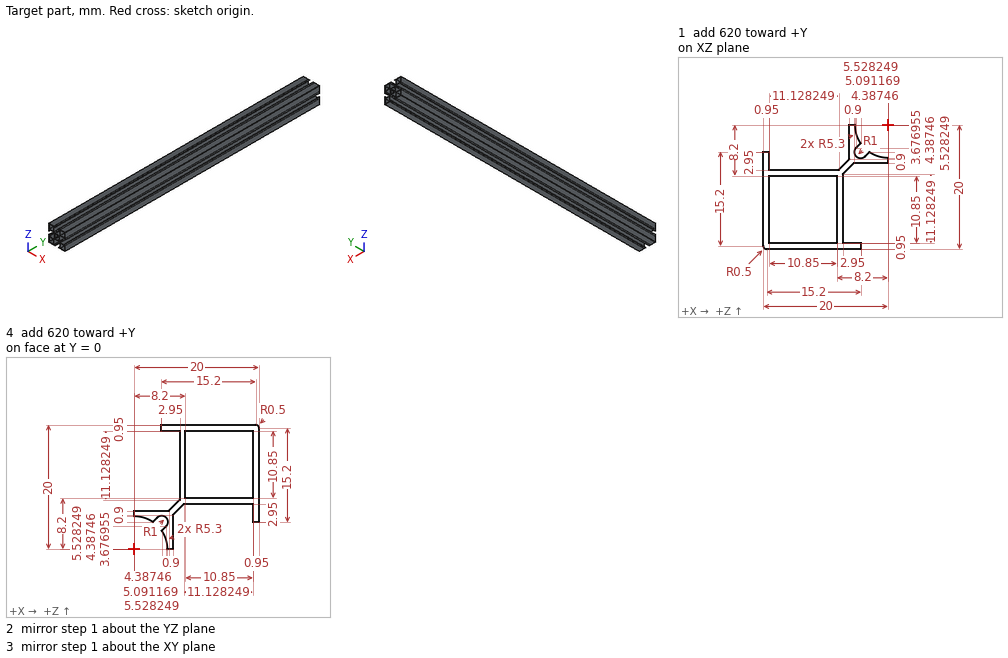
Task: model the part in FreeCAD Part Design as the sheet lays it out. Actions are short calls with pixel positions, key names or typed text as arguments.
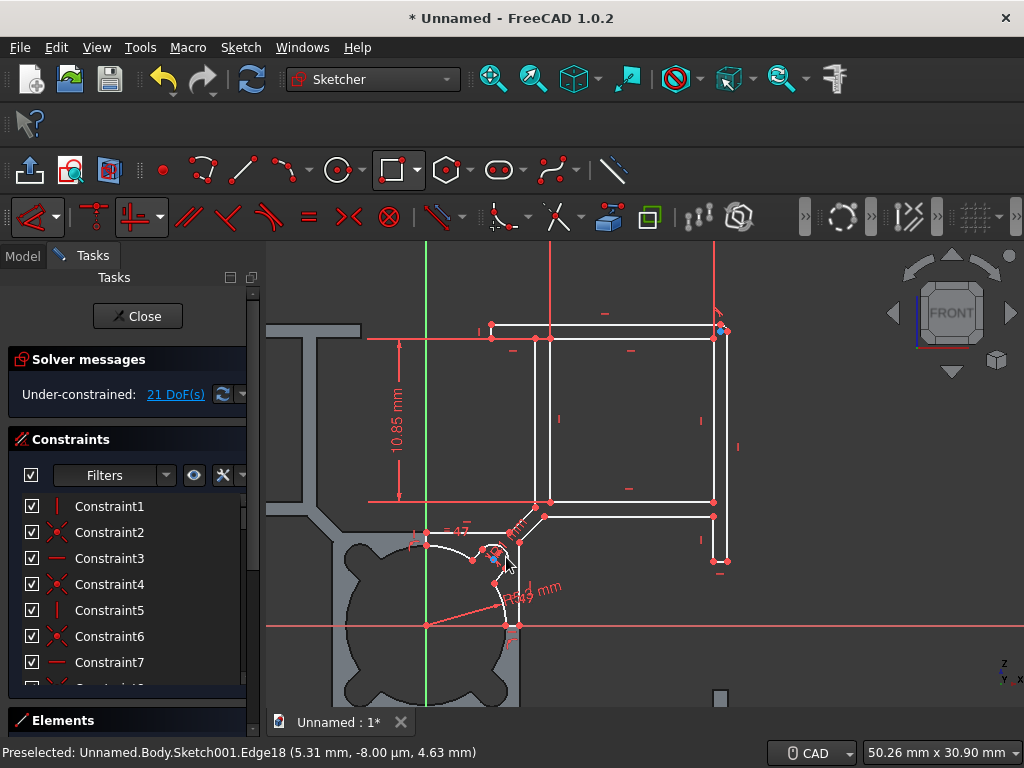
scroll(725, 327, up, 9)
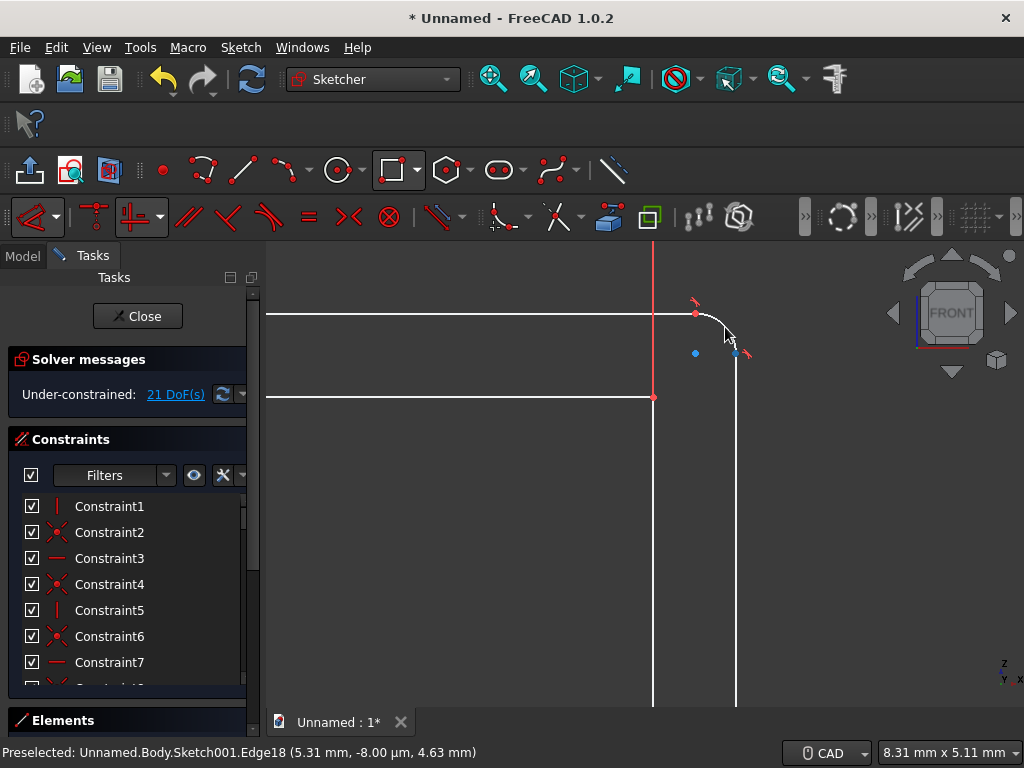
click(724, 325)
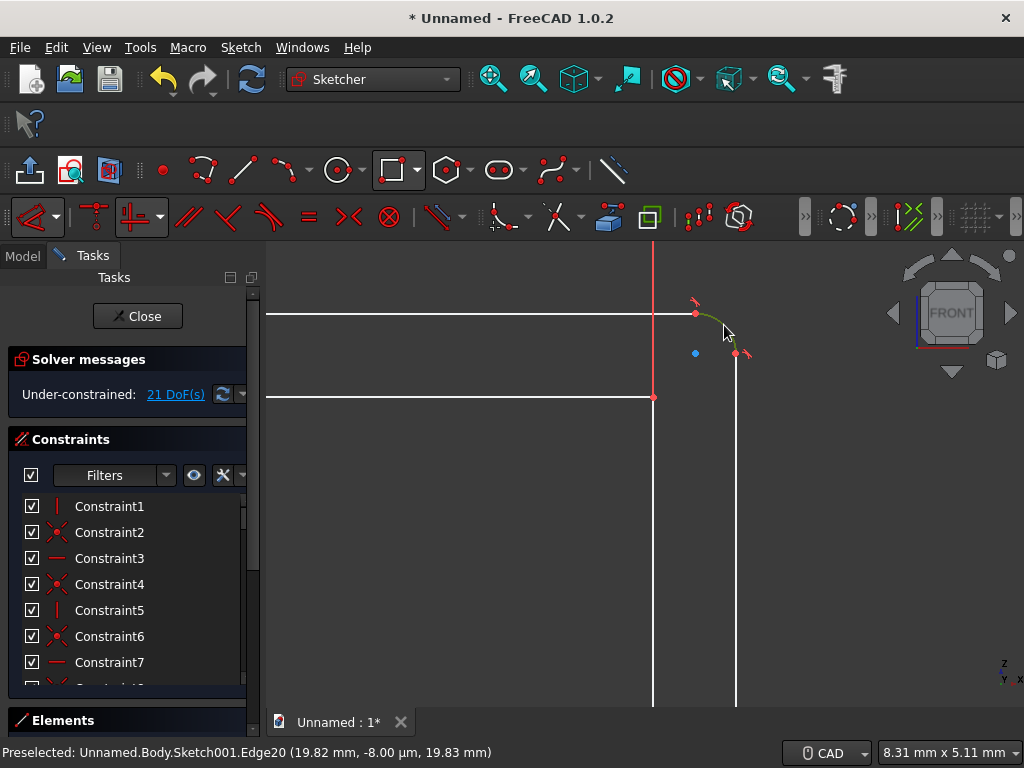
key(k)
key(r)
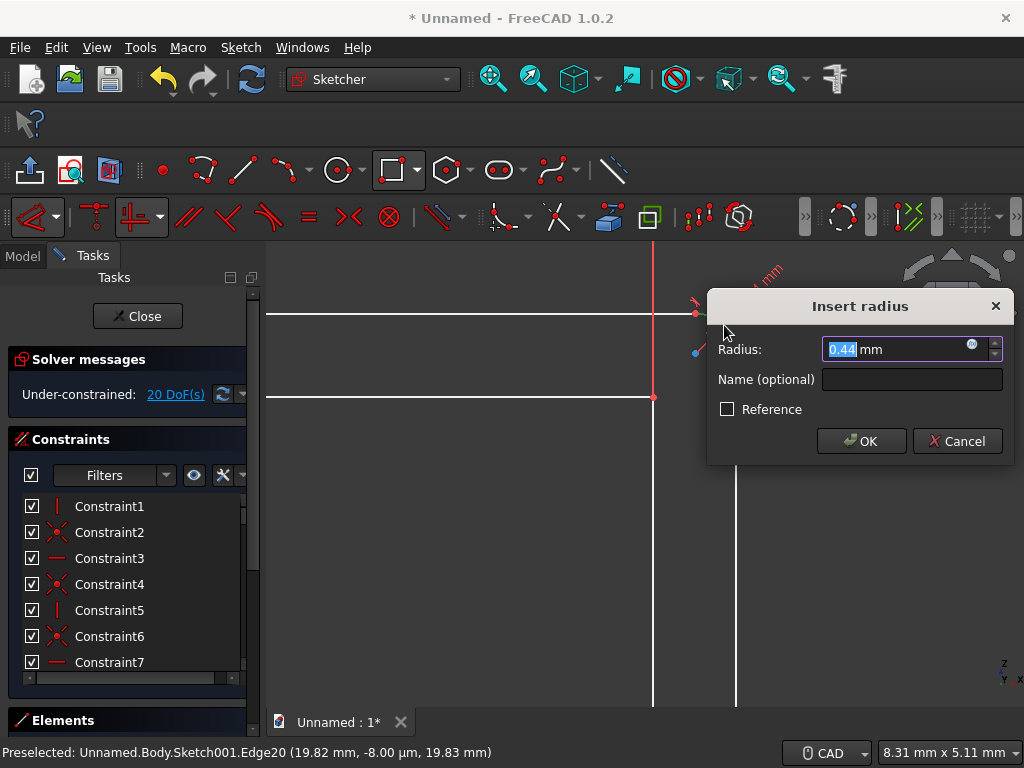
text(0.5)
key(Return)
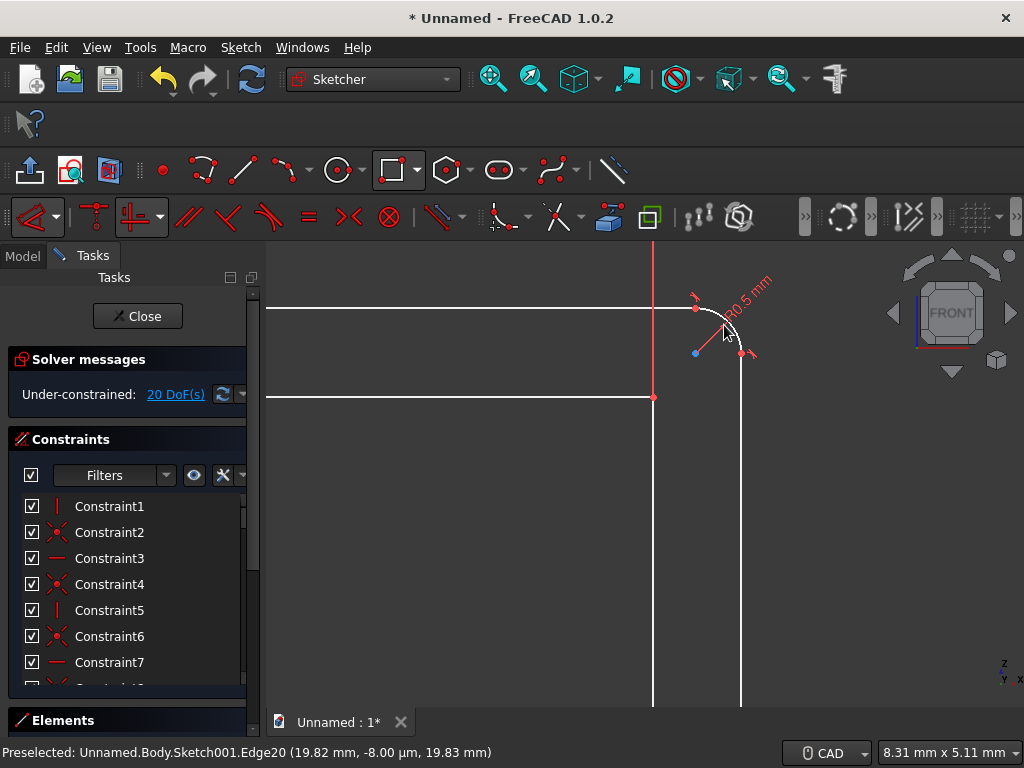
scroll(725, 326, down, 9)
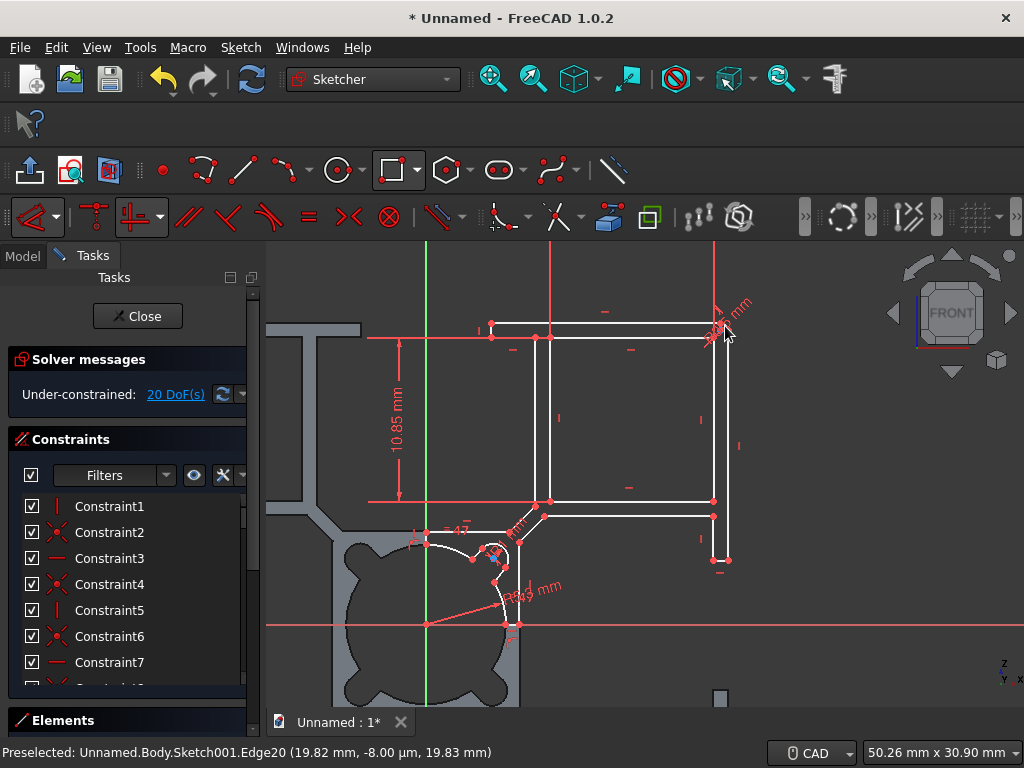
scroll(515, 625, up, 7)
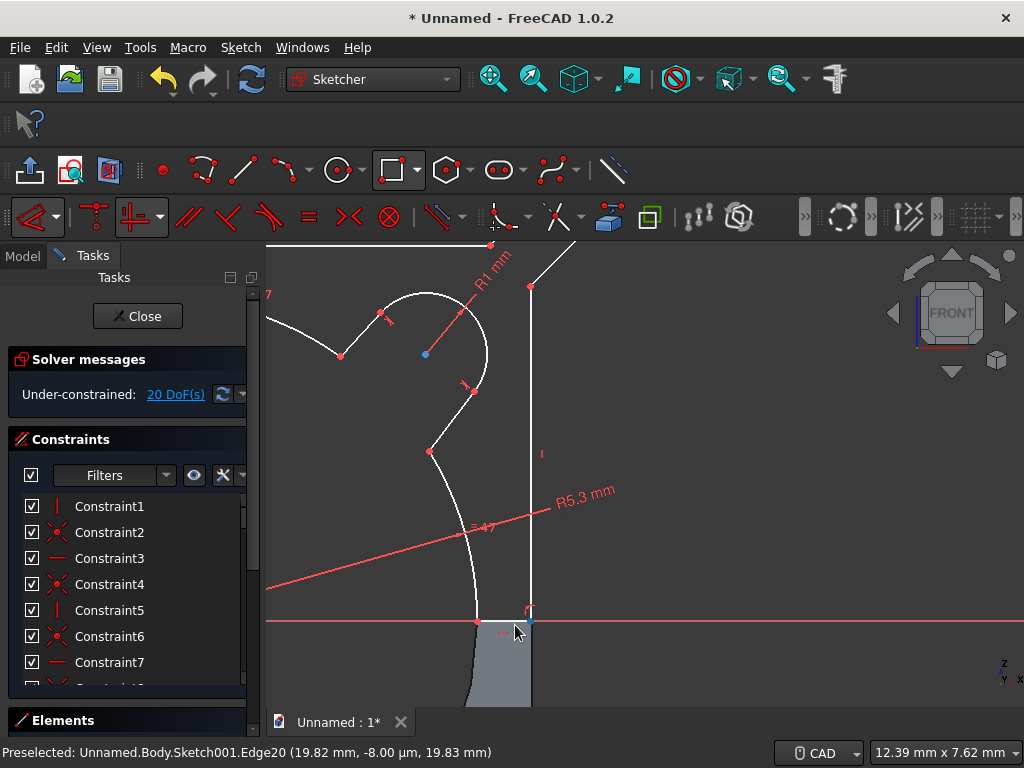
click(515, 621)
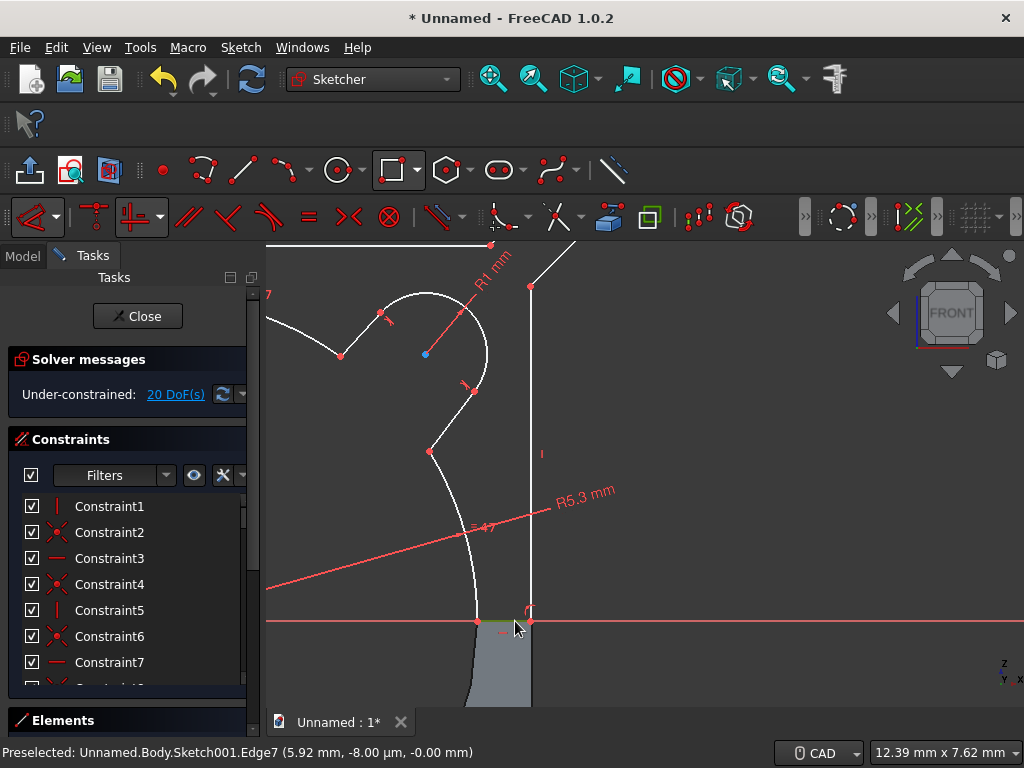
key(l)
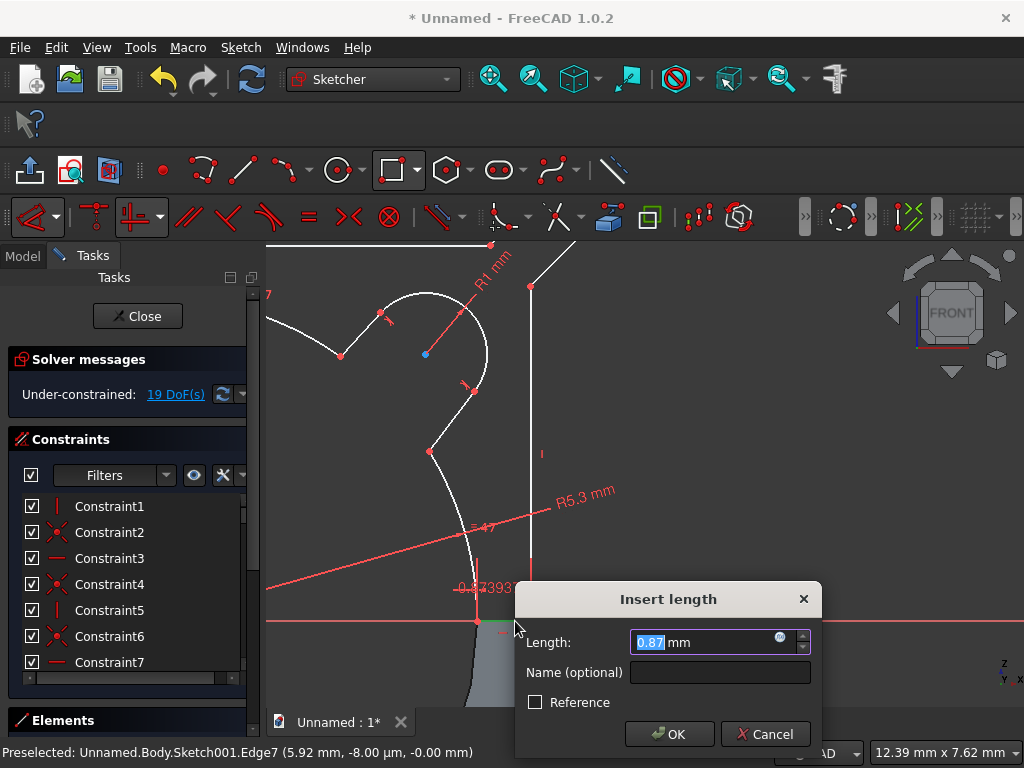
text(0.9)
key(Return)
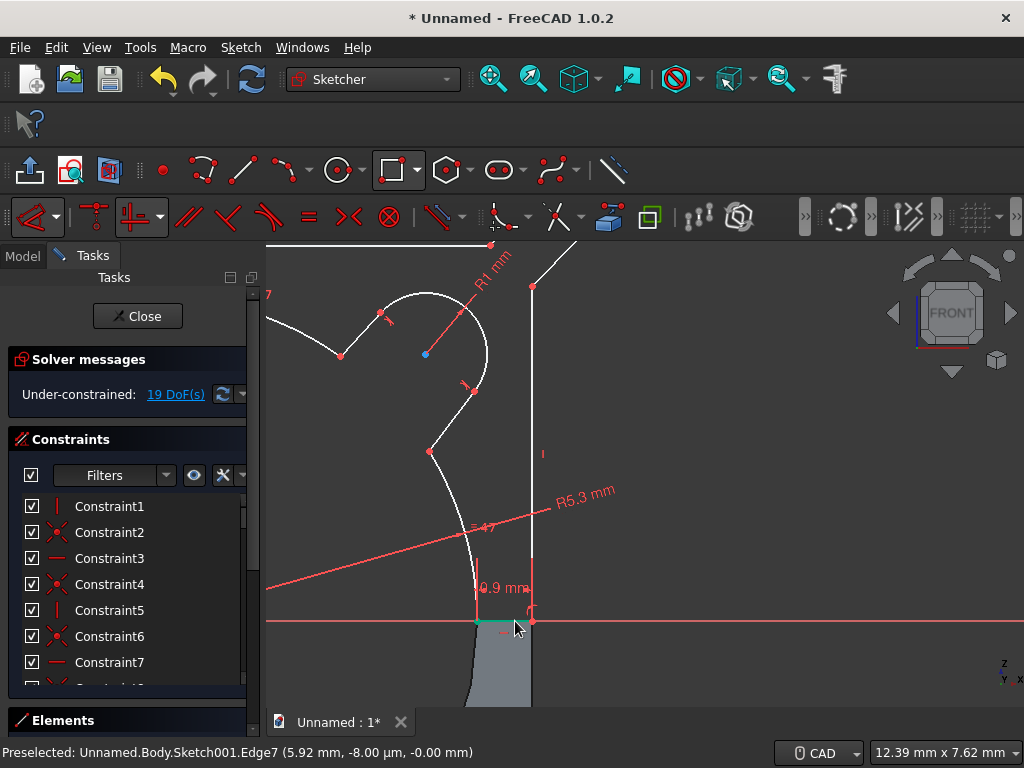
scroll(515, 626, down, 7)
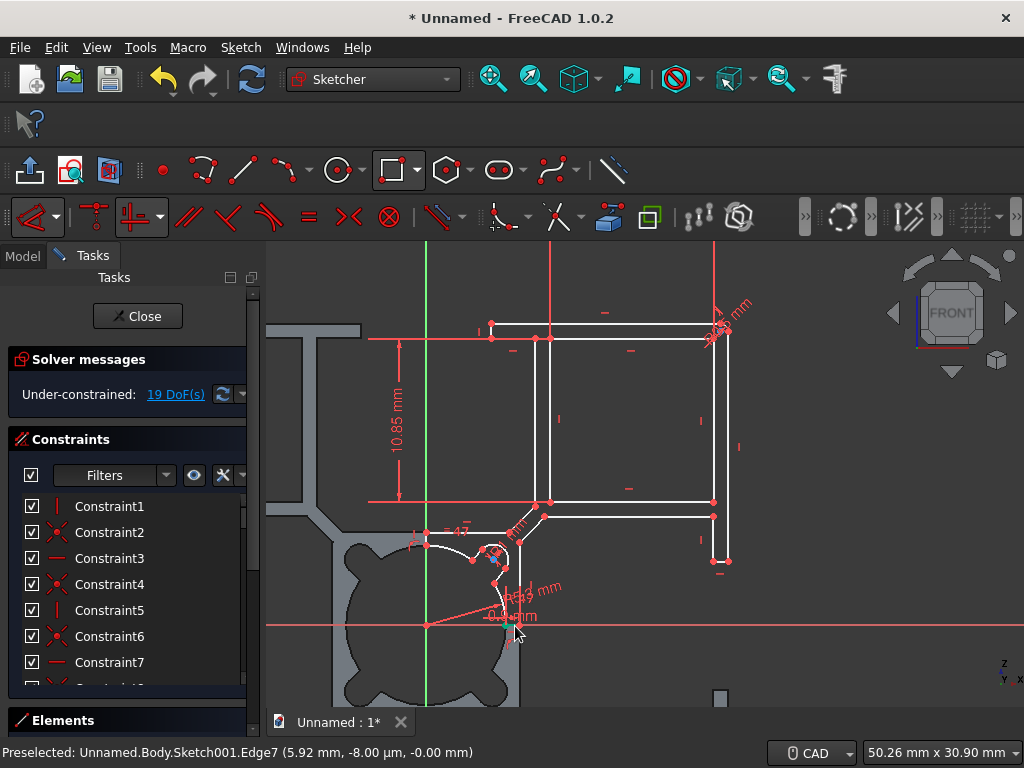
scroll(426, 542, up, 7)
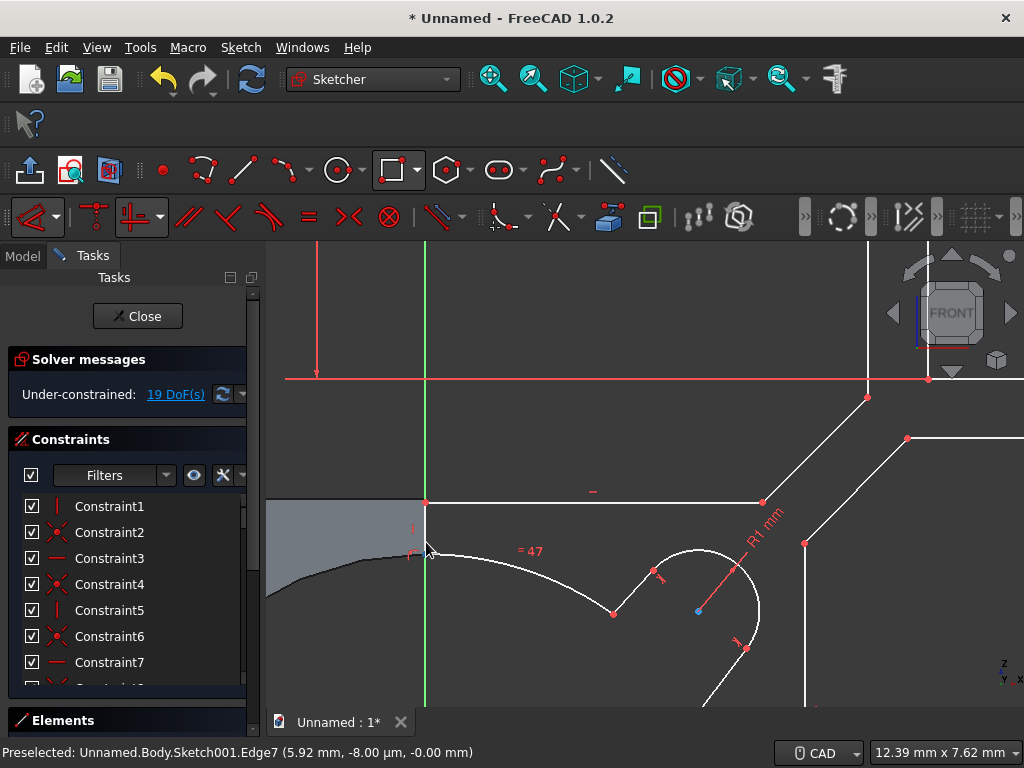
click(425, 539)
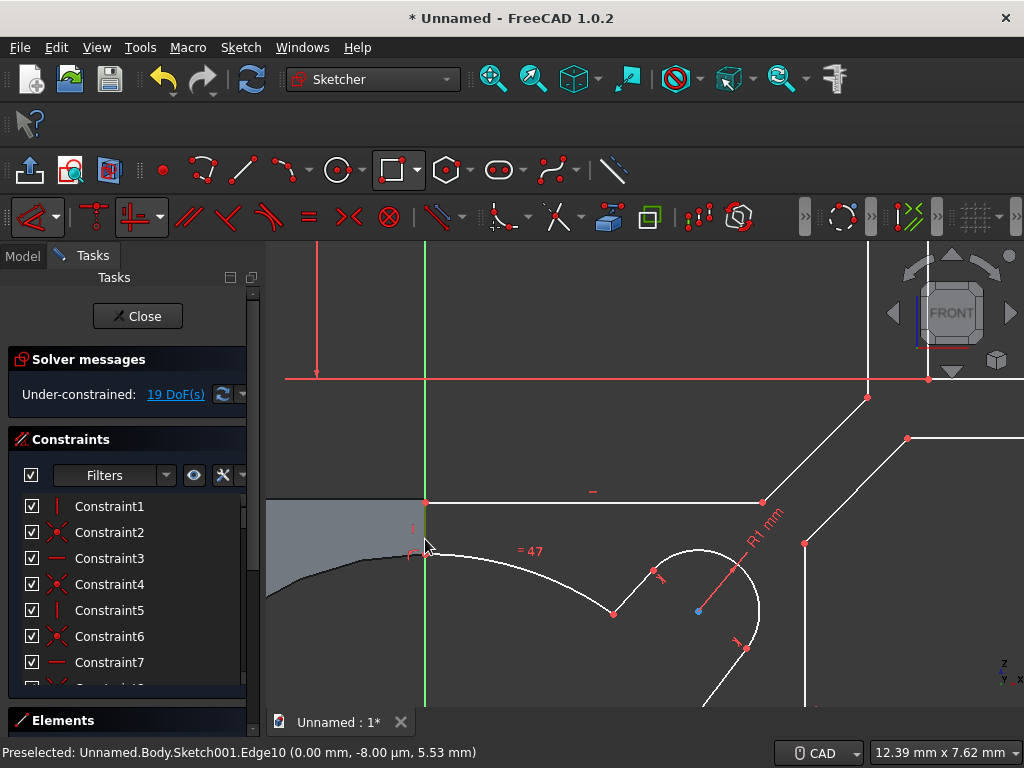
key(i)